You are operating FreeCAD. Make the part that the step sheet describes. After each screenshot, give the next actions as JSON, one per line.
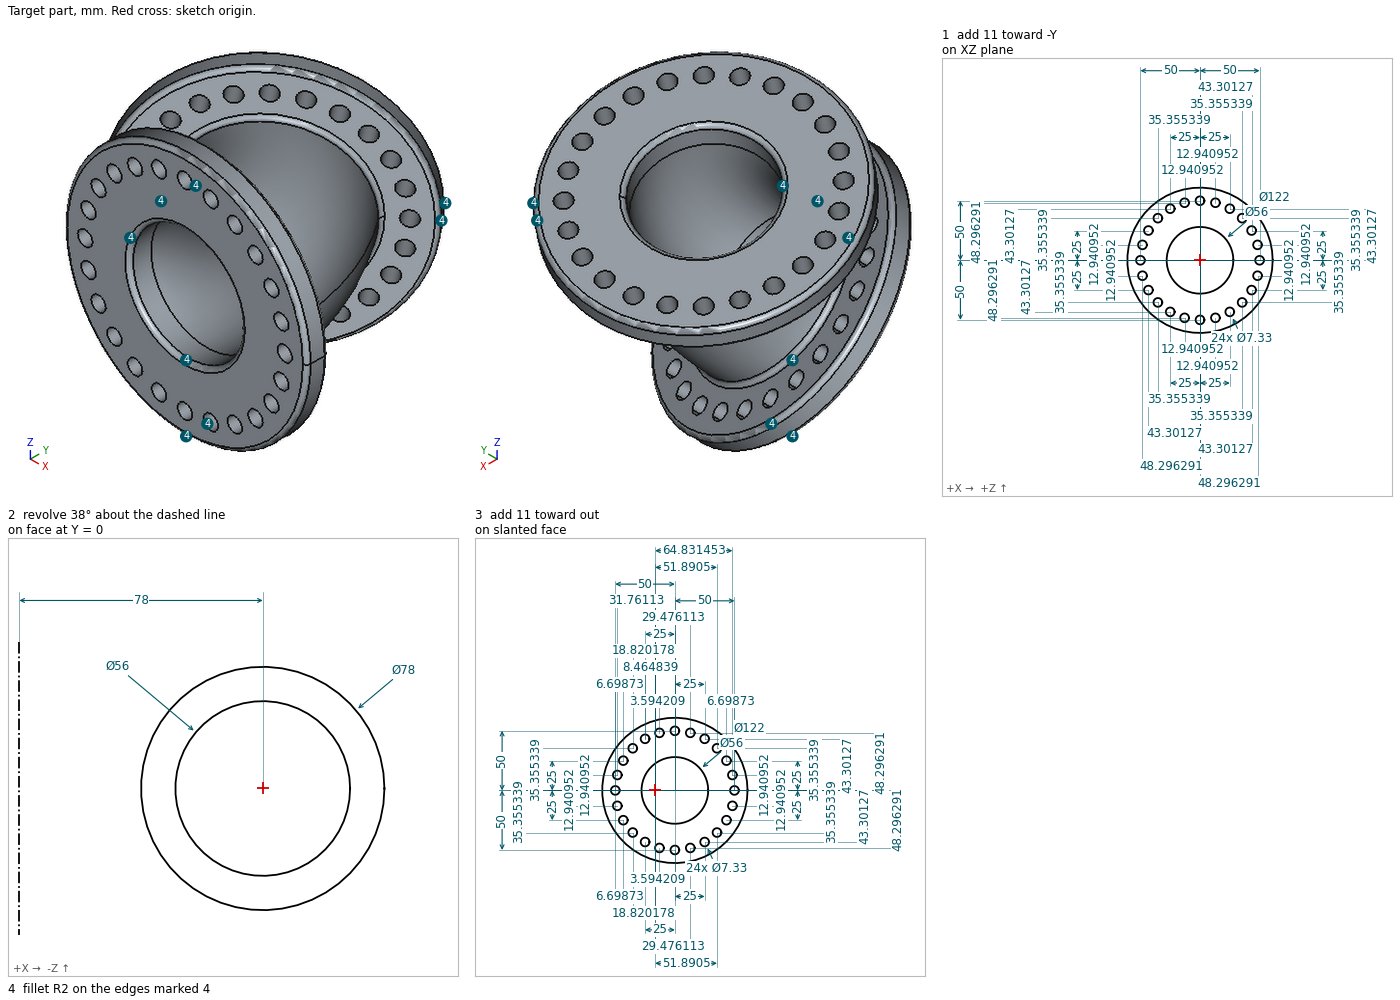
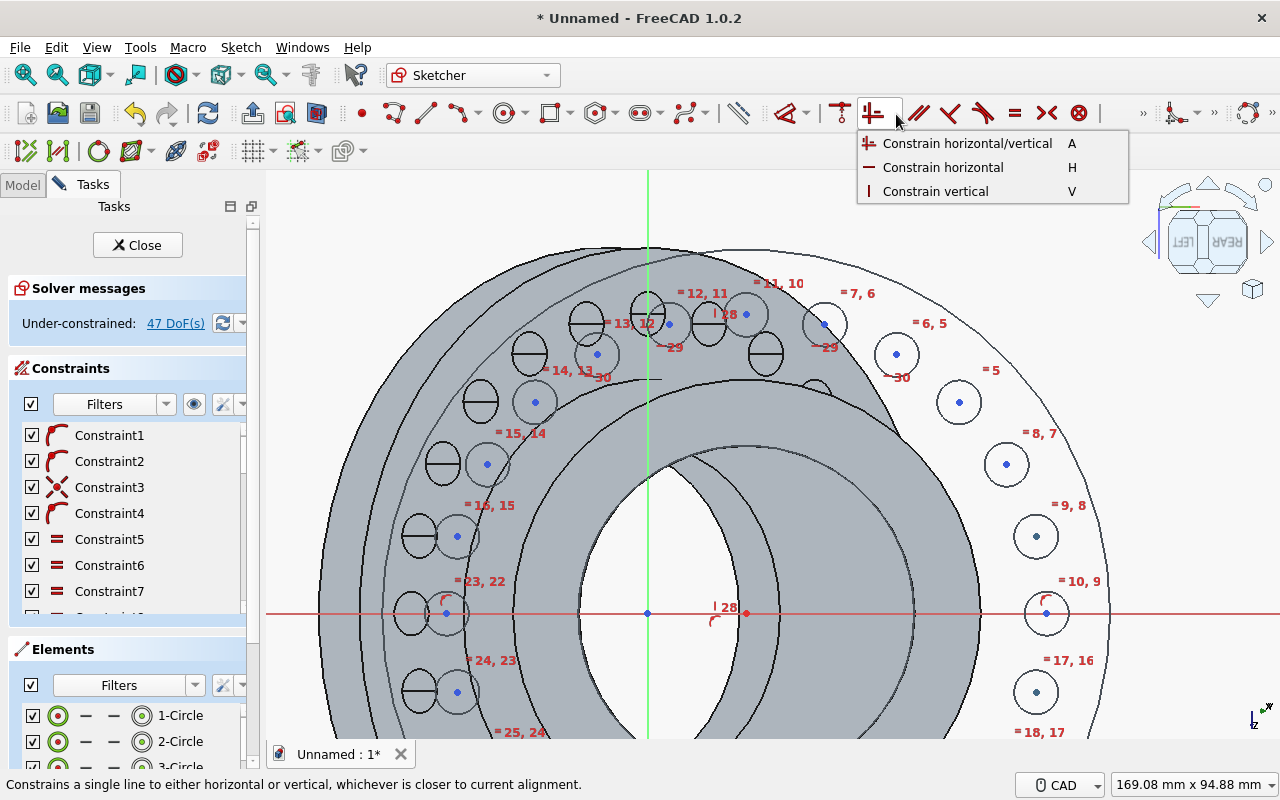
{"action": "left_click", "coordinate": [993, 191]}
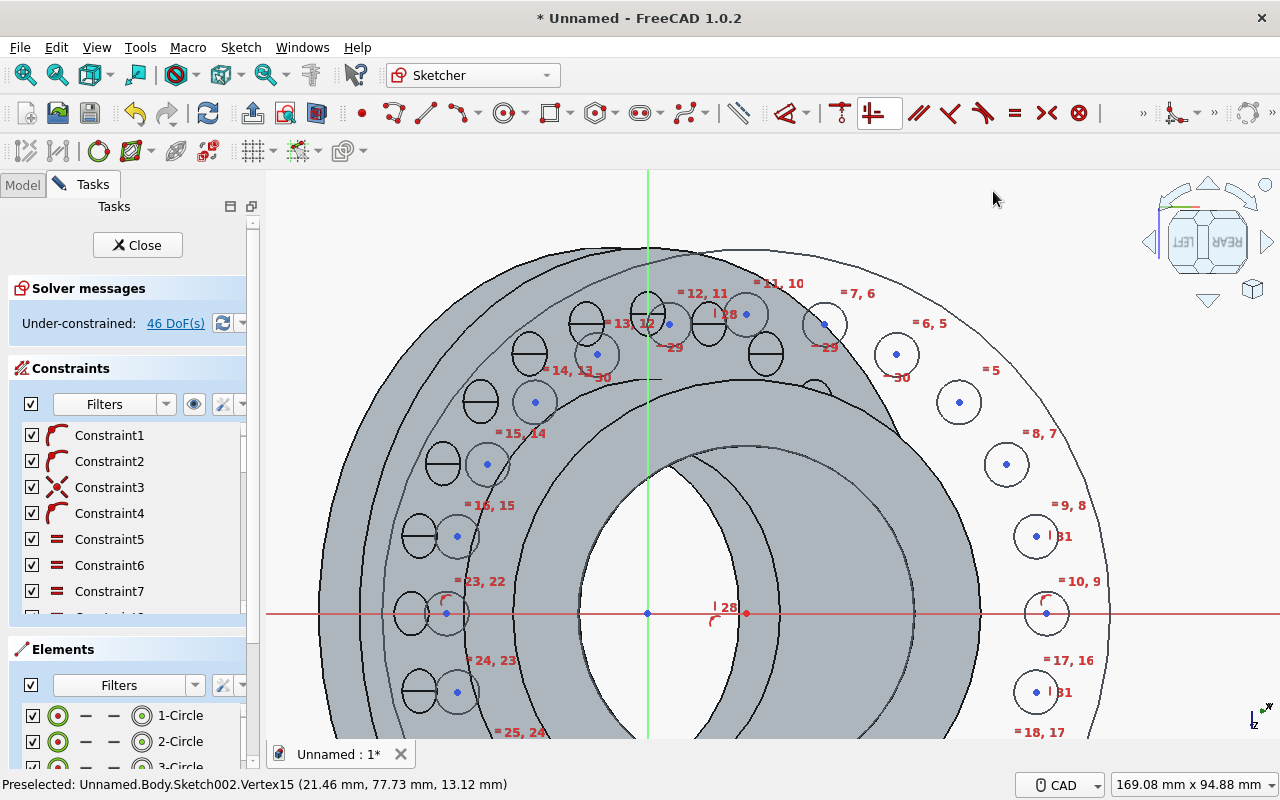
{"action": "left_click", "coordinate": [1007, 465]}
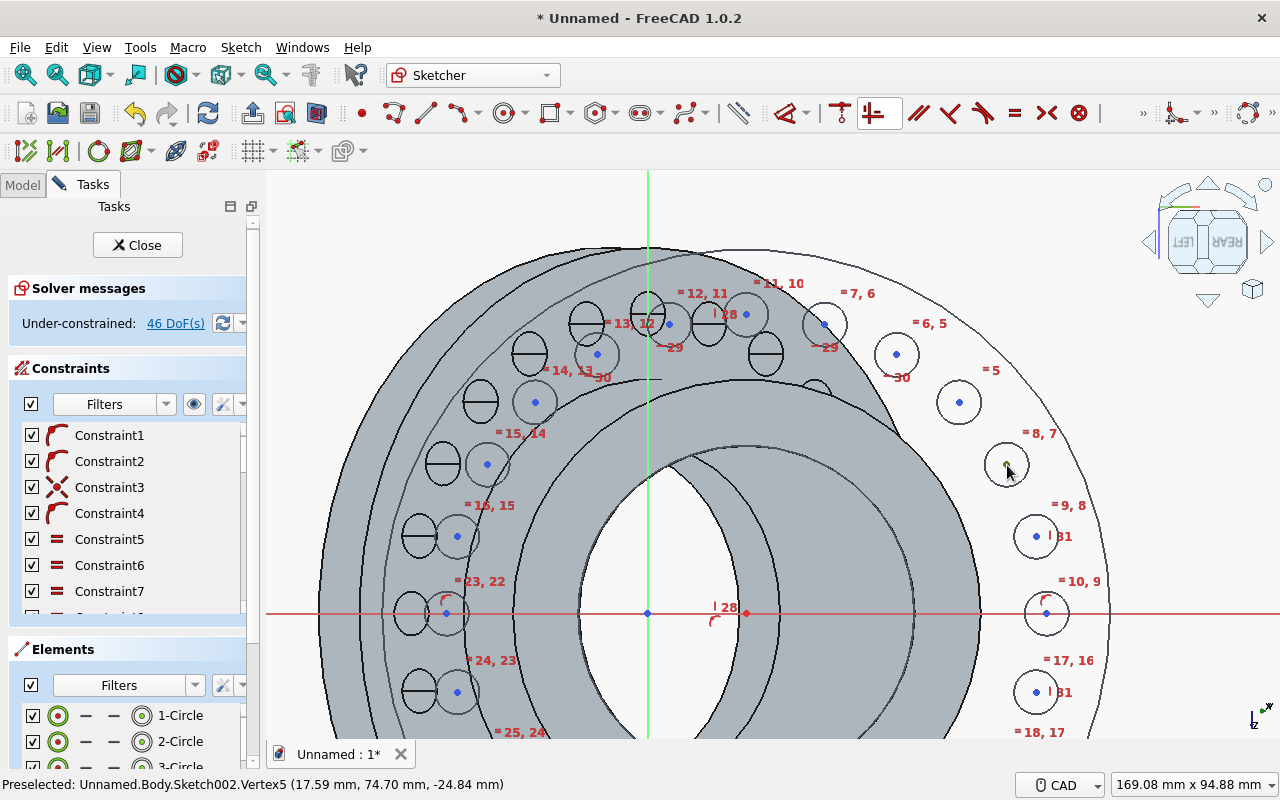
{"action": "scroll", "coordinate": [670, 325], "scroll_direction": "down", "scroll_amount": 4}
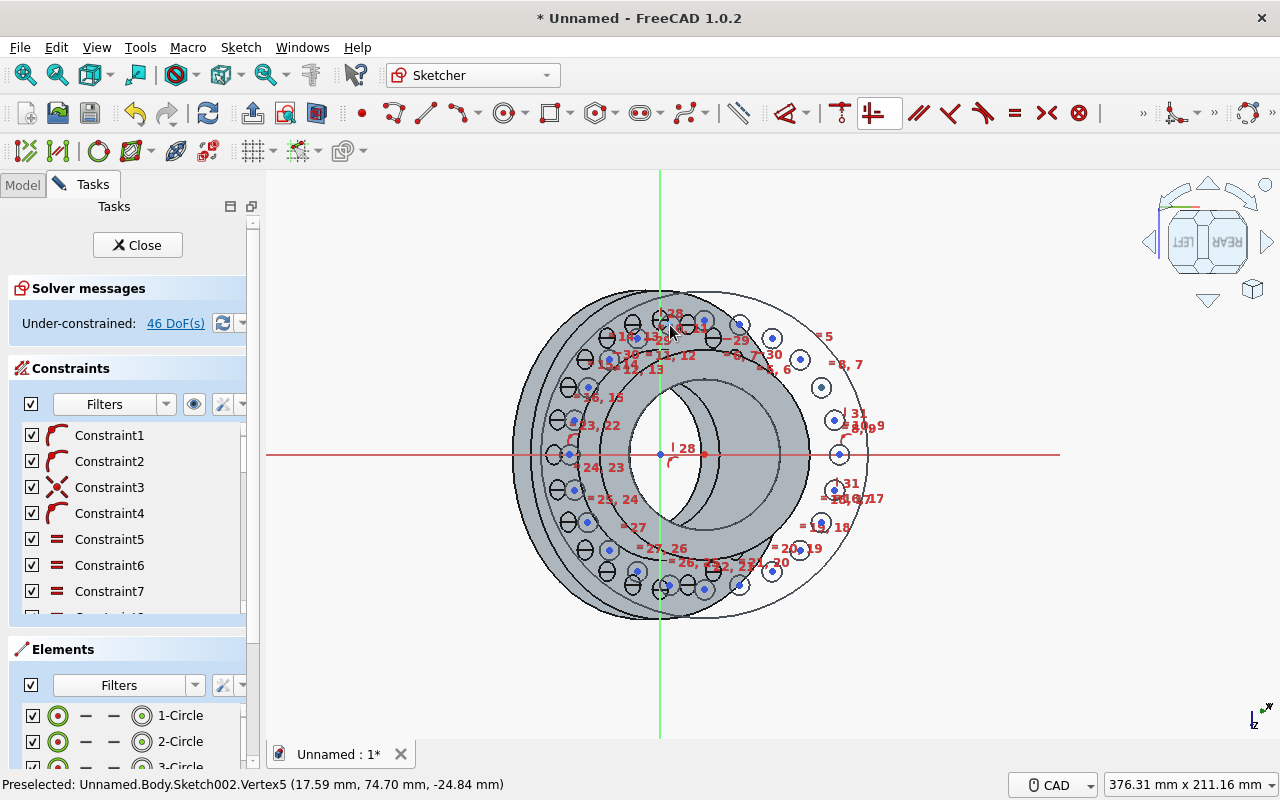
{"action": "left_click", "coordinate": [821, 523]}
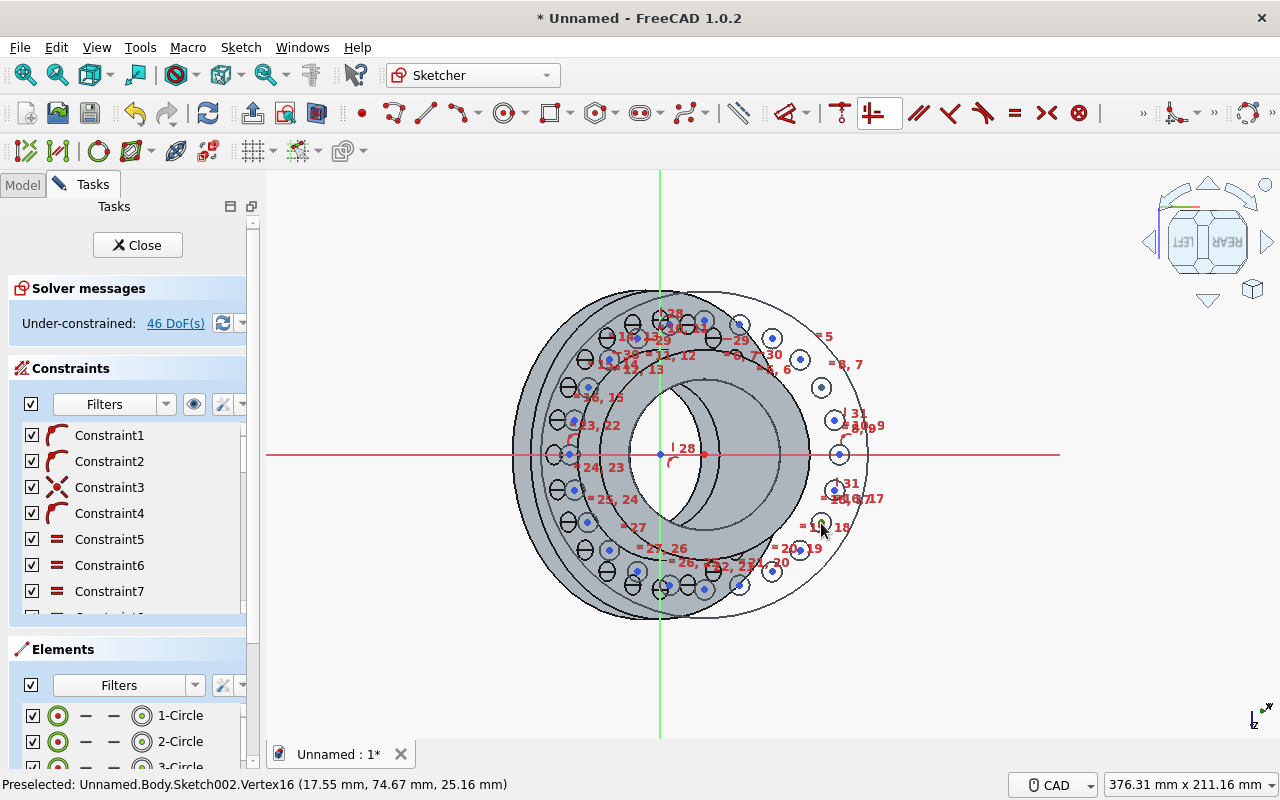
{"action": "key", "text": "v"}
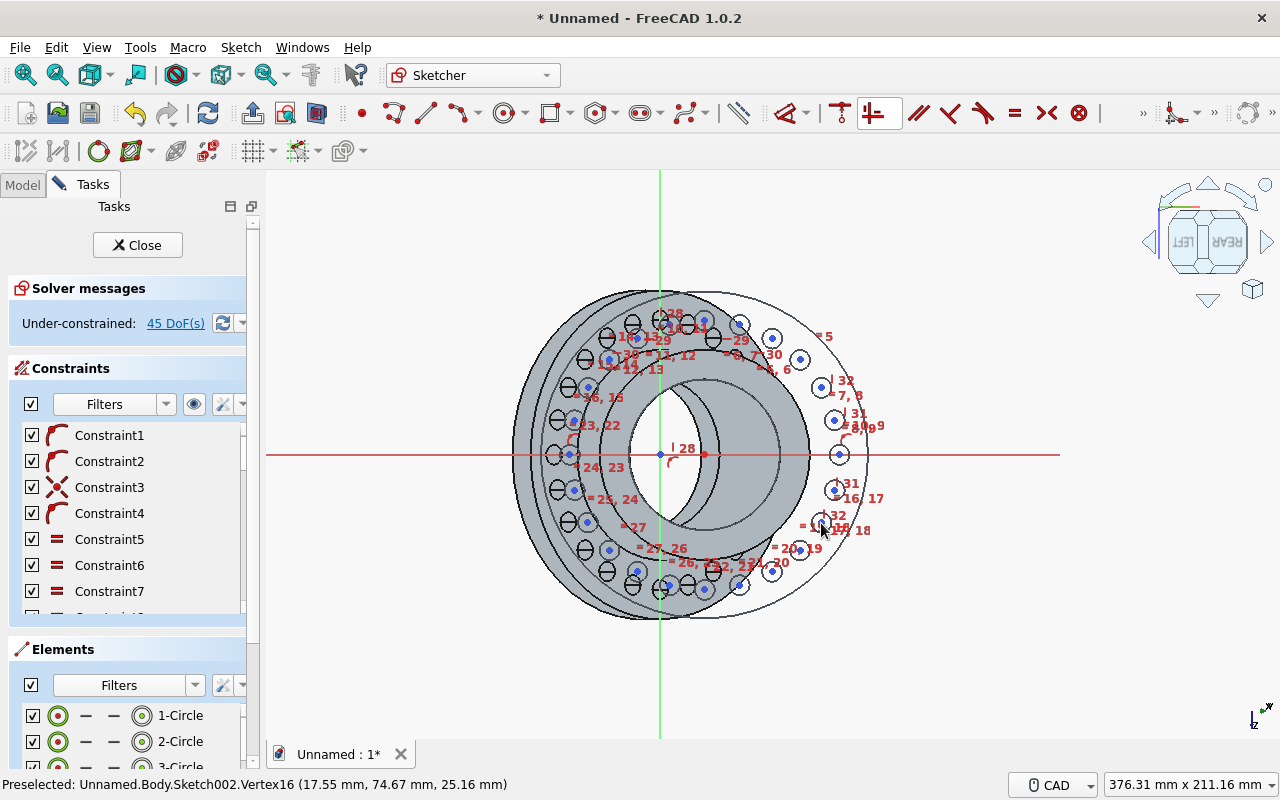
{"action": "left_click", "coordinate": [704, 455]}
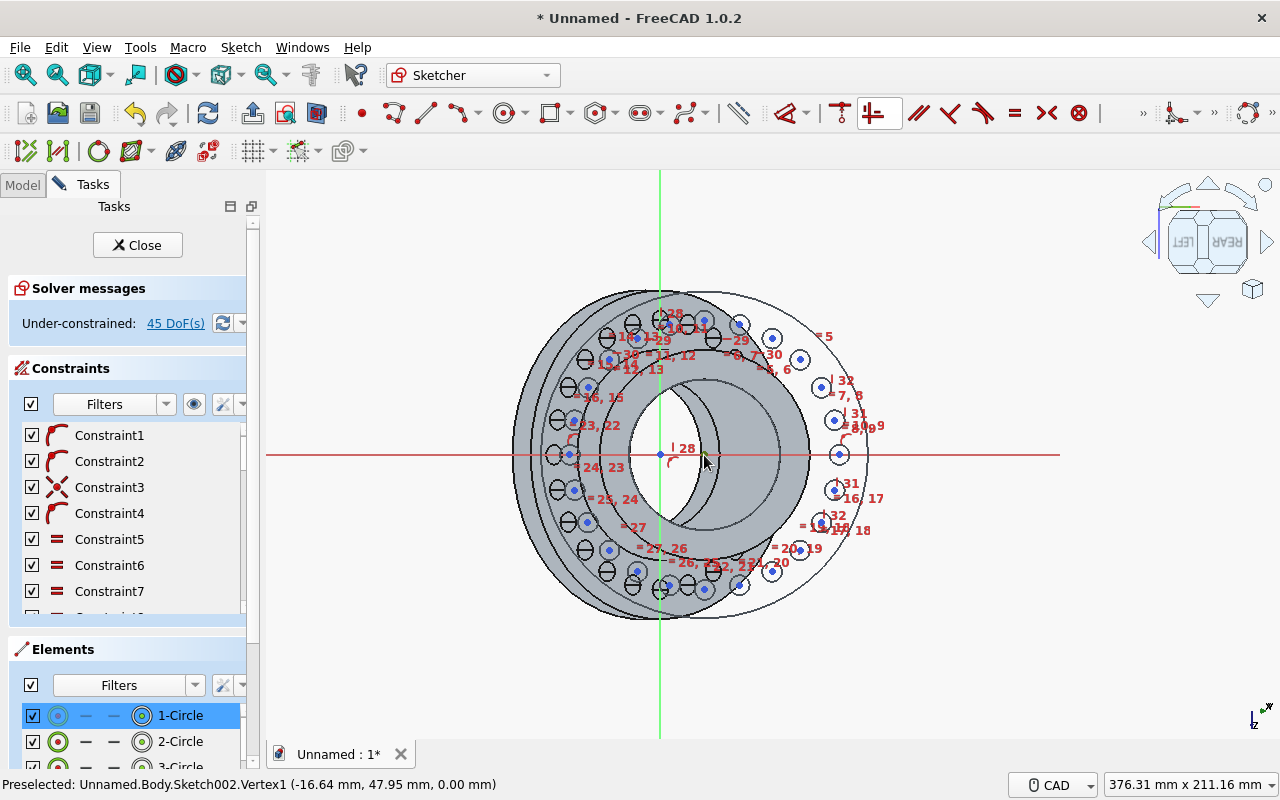
{"action": "left_click", "coordinate": [705, 590]}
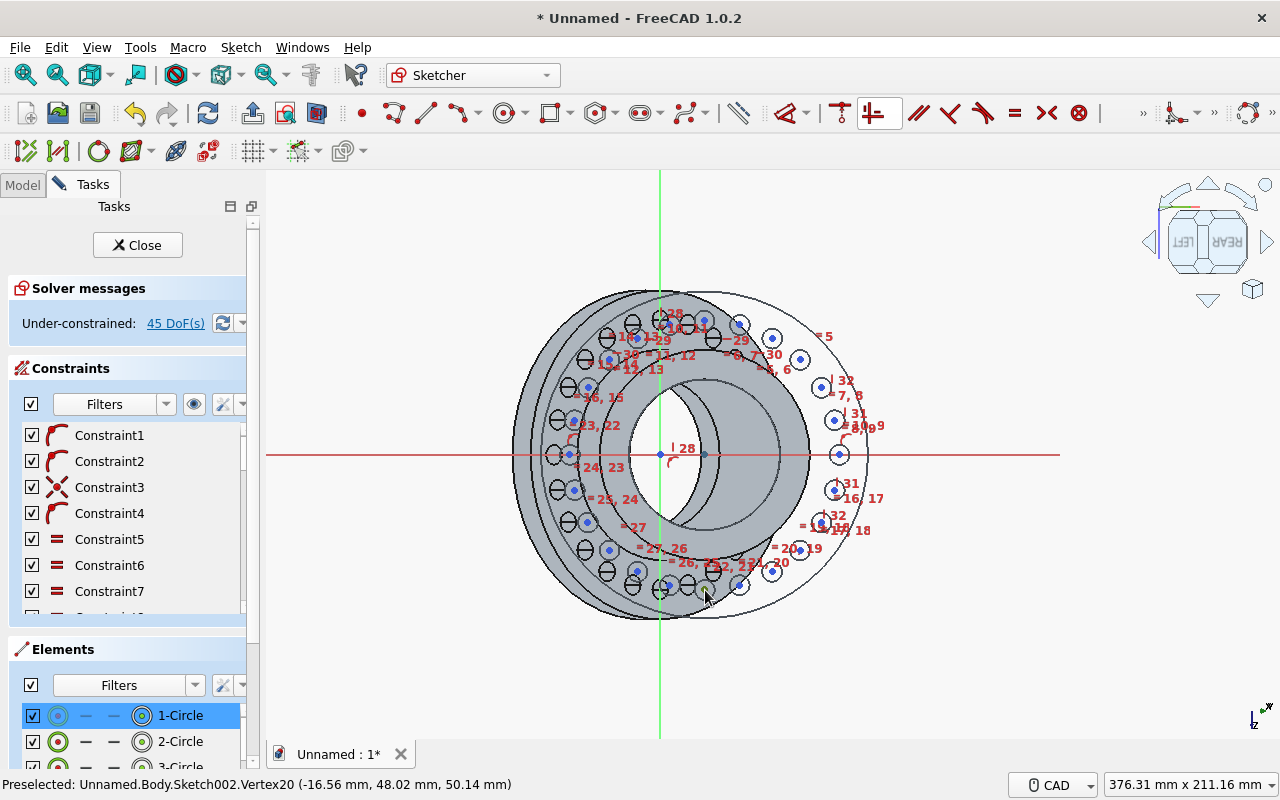
{"action": "key", "text": "v"}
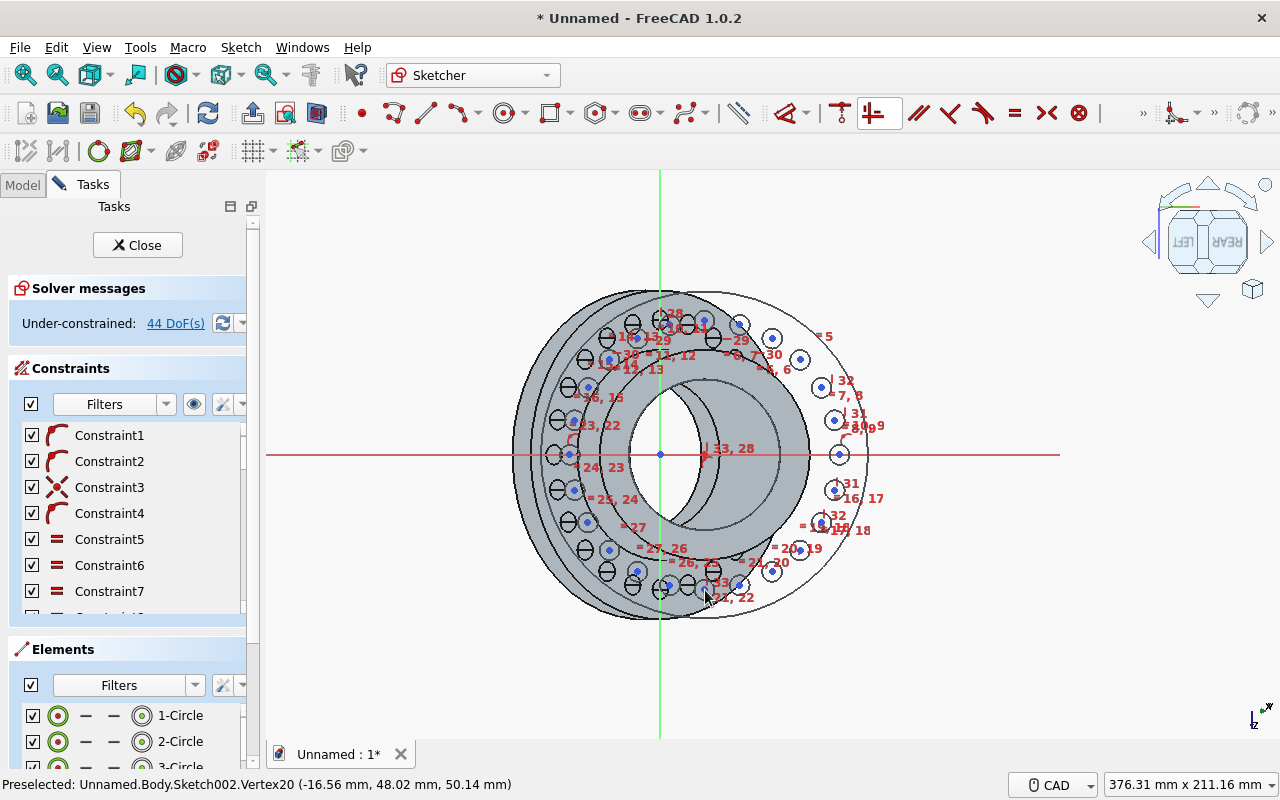
{"action": "left_click", "coordinate": [575, 420]}